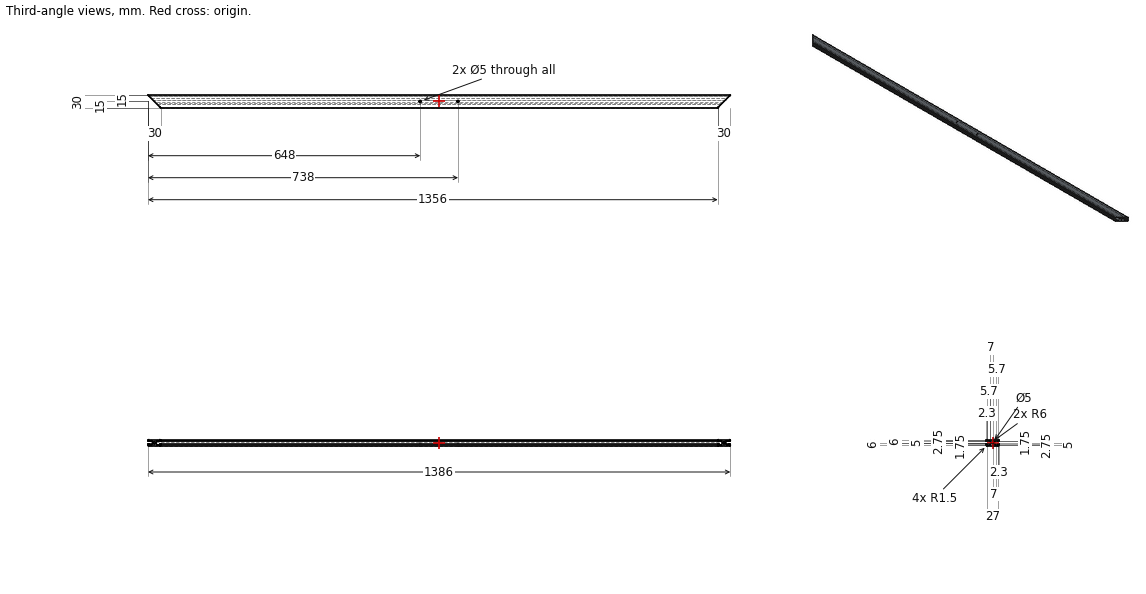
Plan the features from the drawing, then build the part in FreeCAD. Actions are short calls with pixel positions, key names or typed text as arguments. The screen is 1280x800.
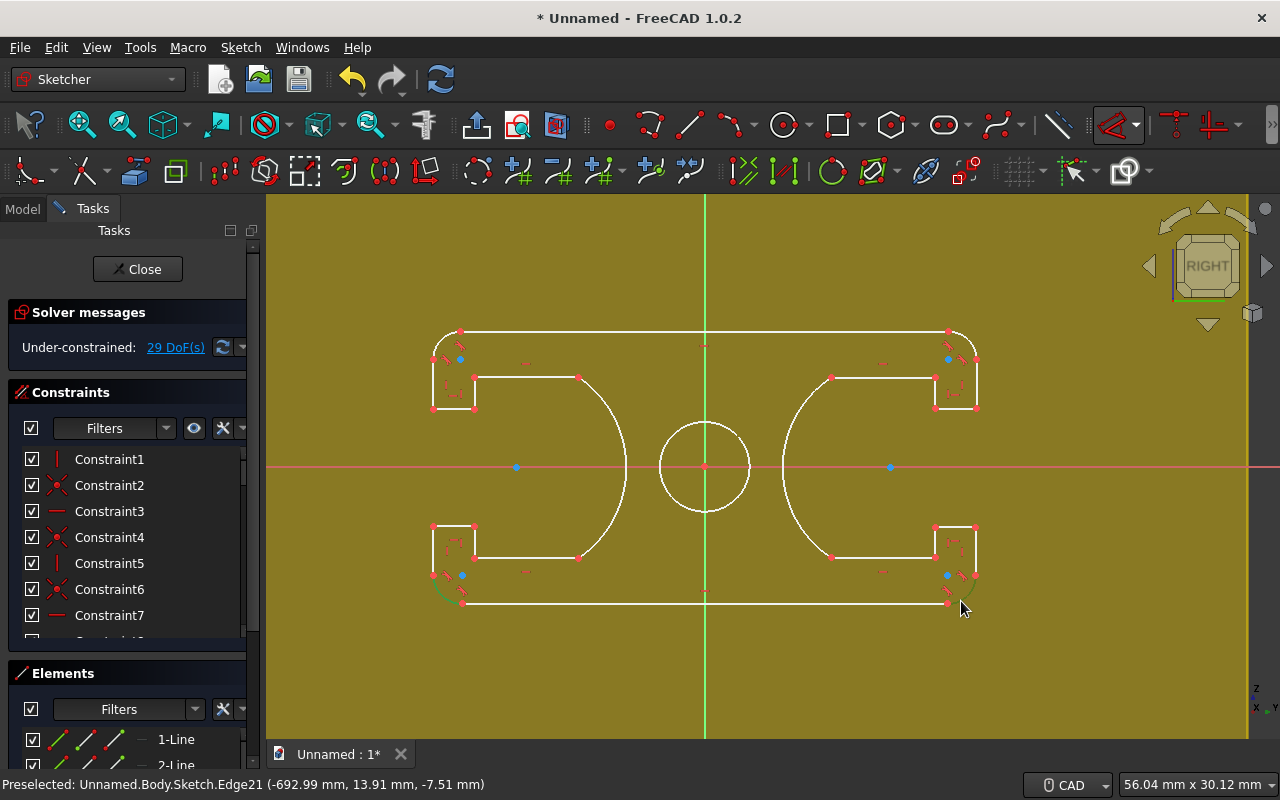
click(973, 347)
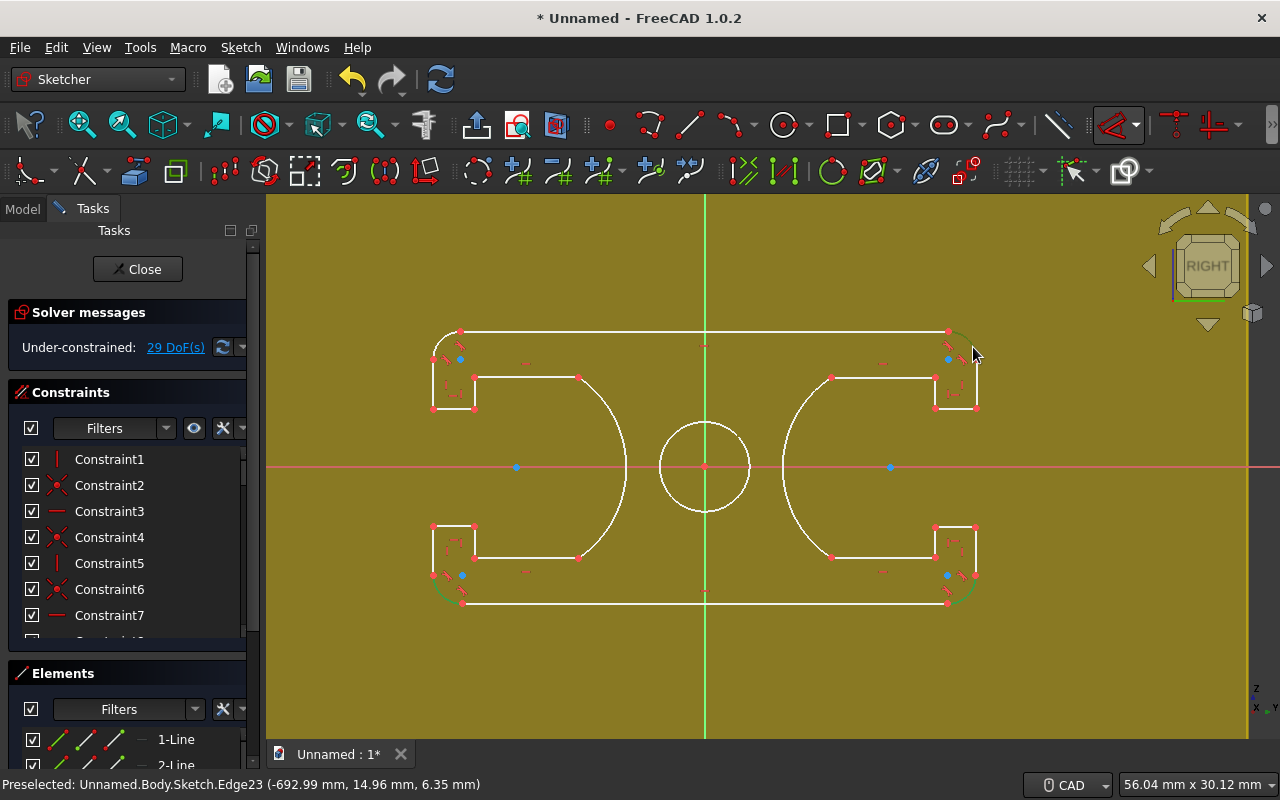
click(448, 335)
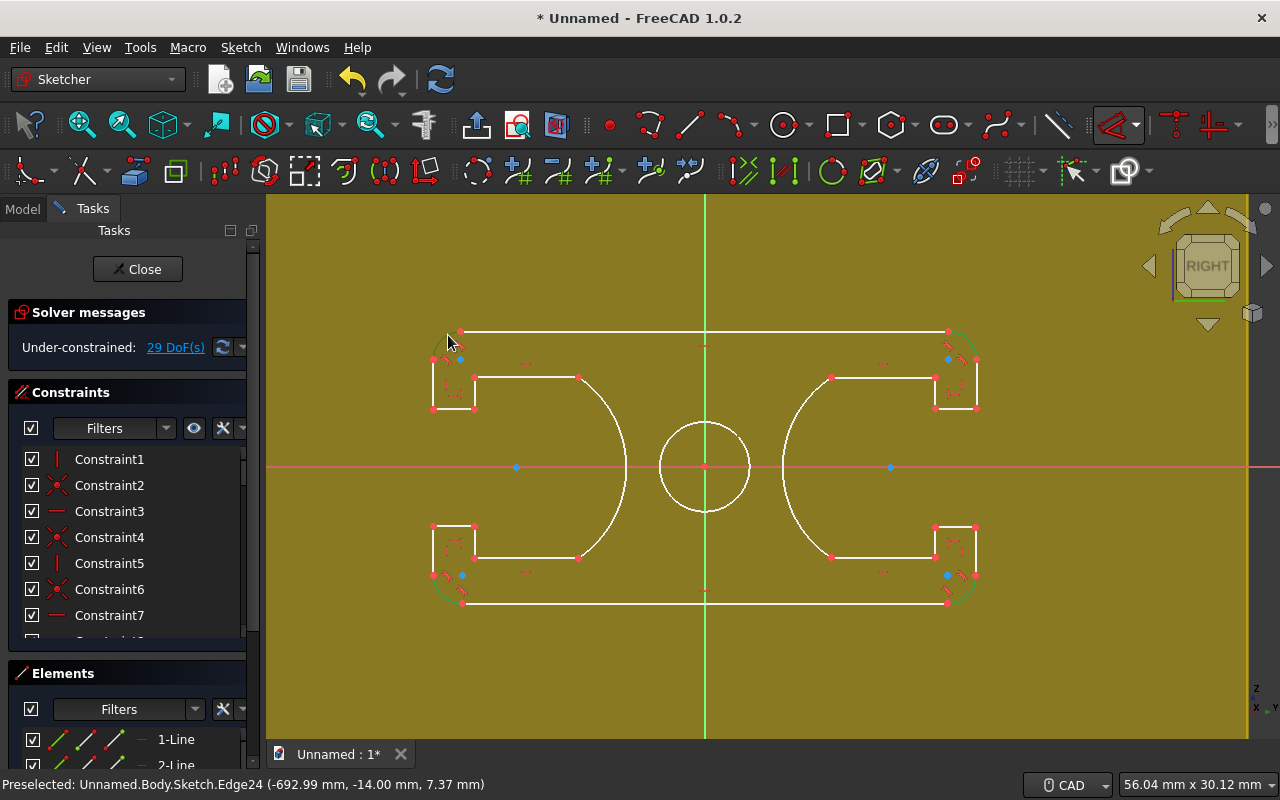
key(e)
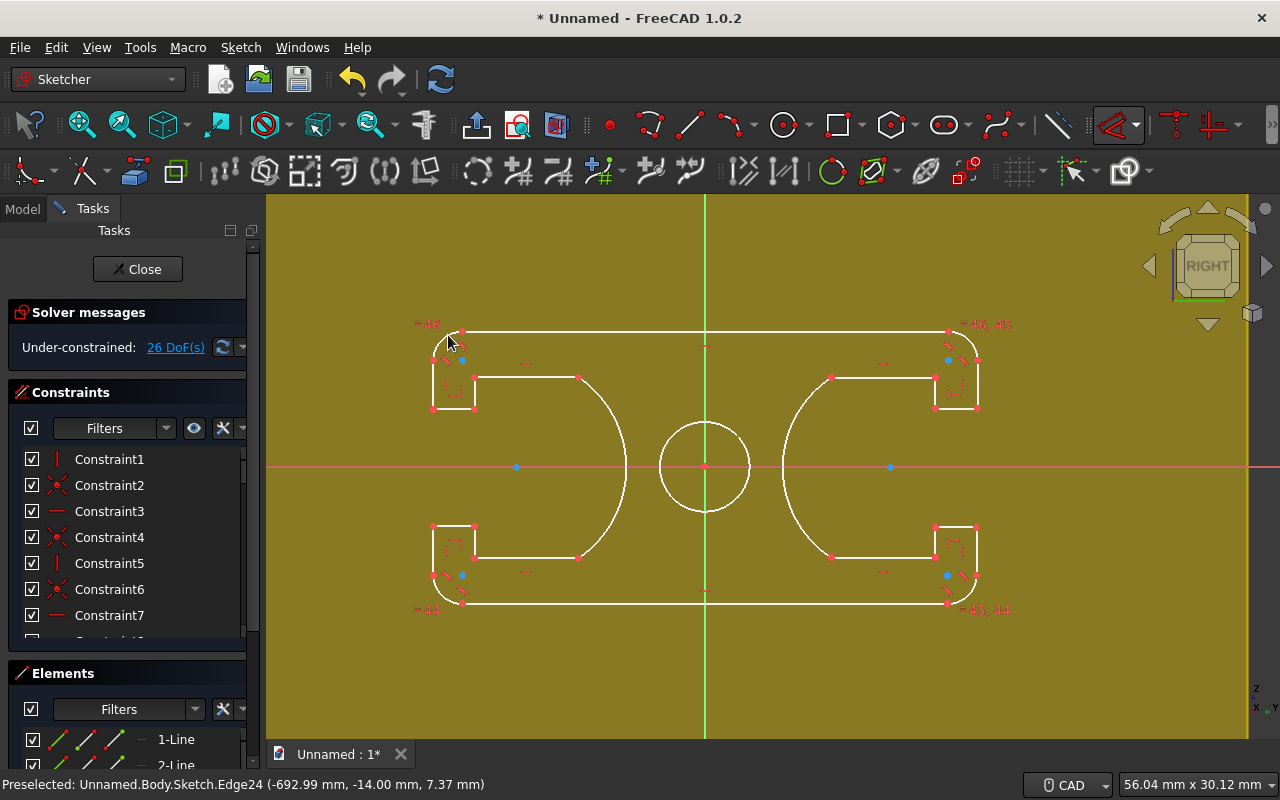
click(618, 509)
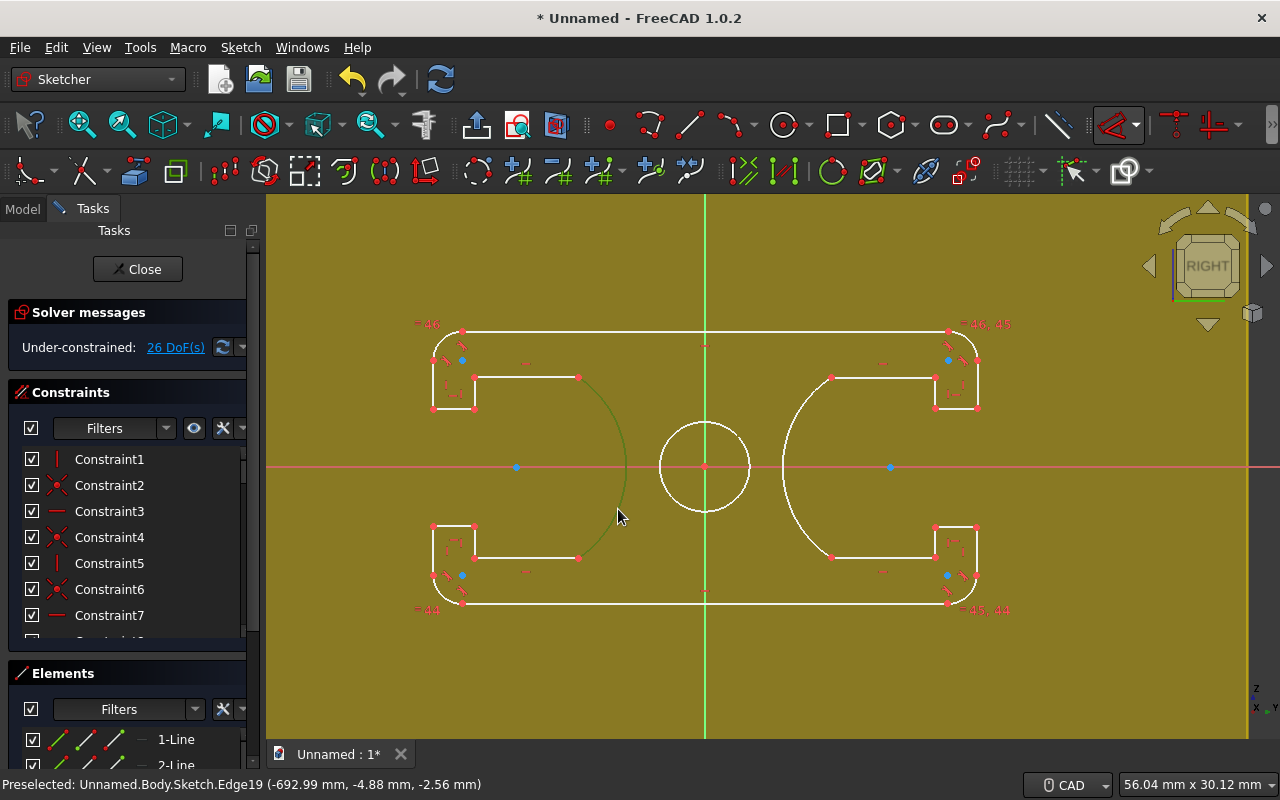
click(791, 426)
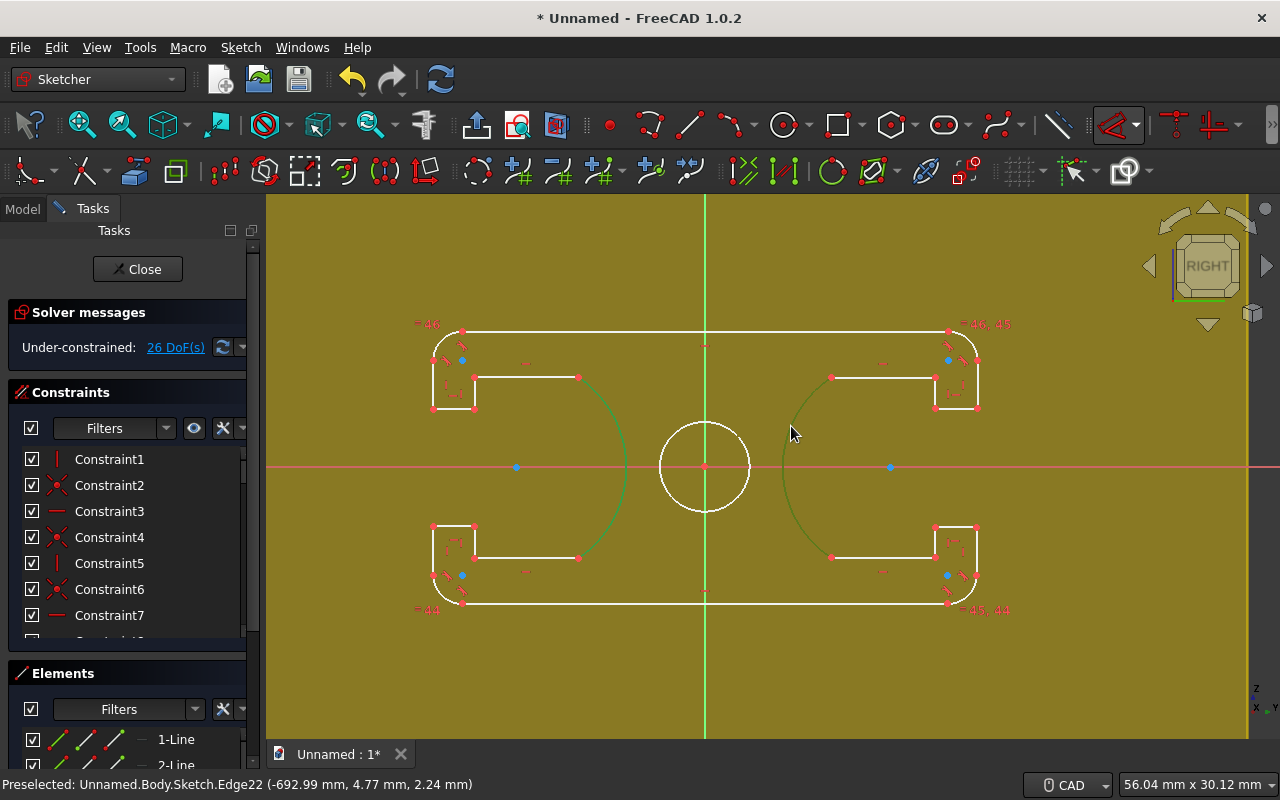
key(e)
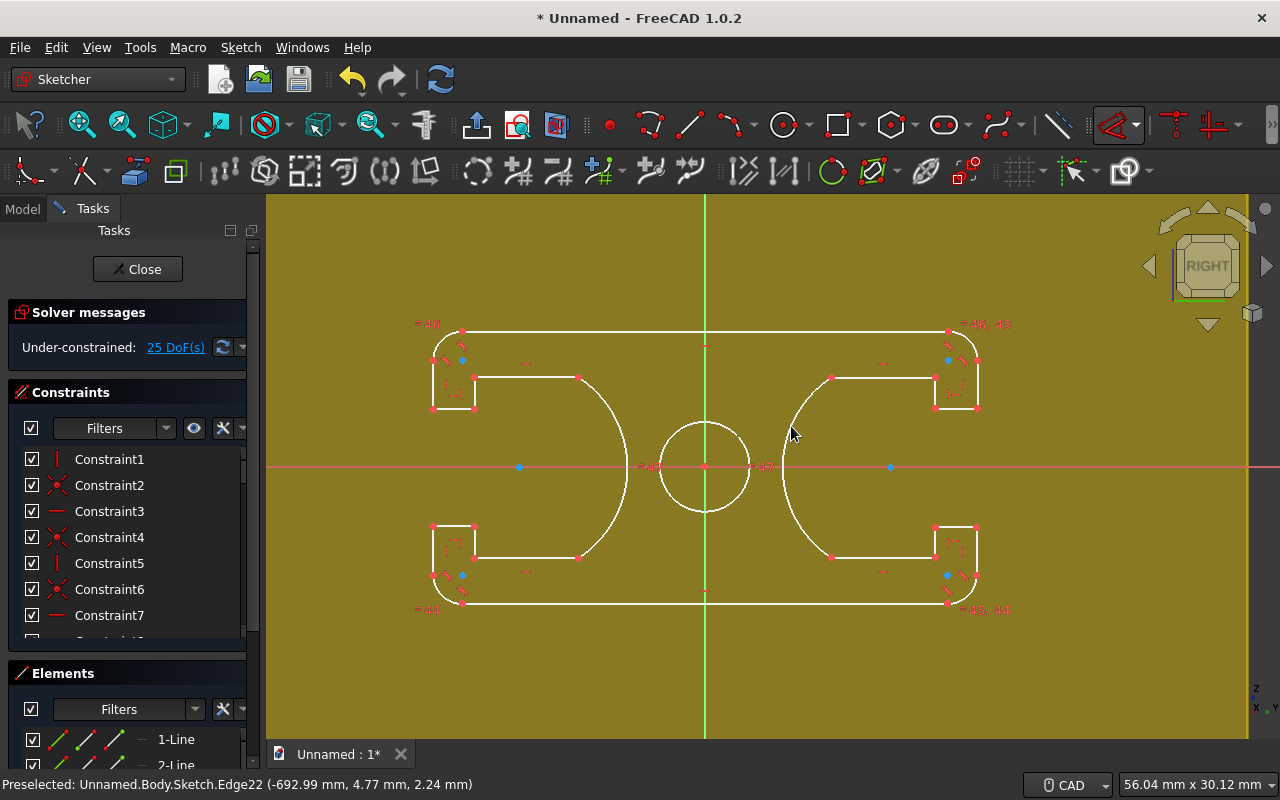
click(519, 468)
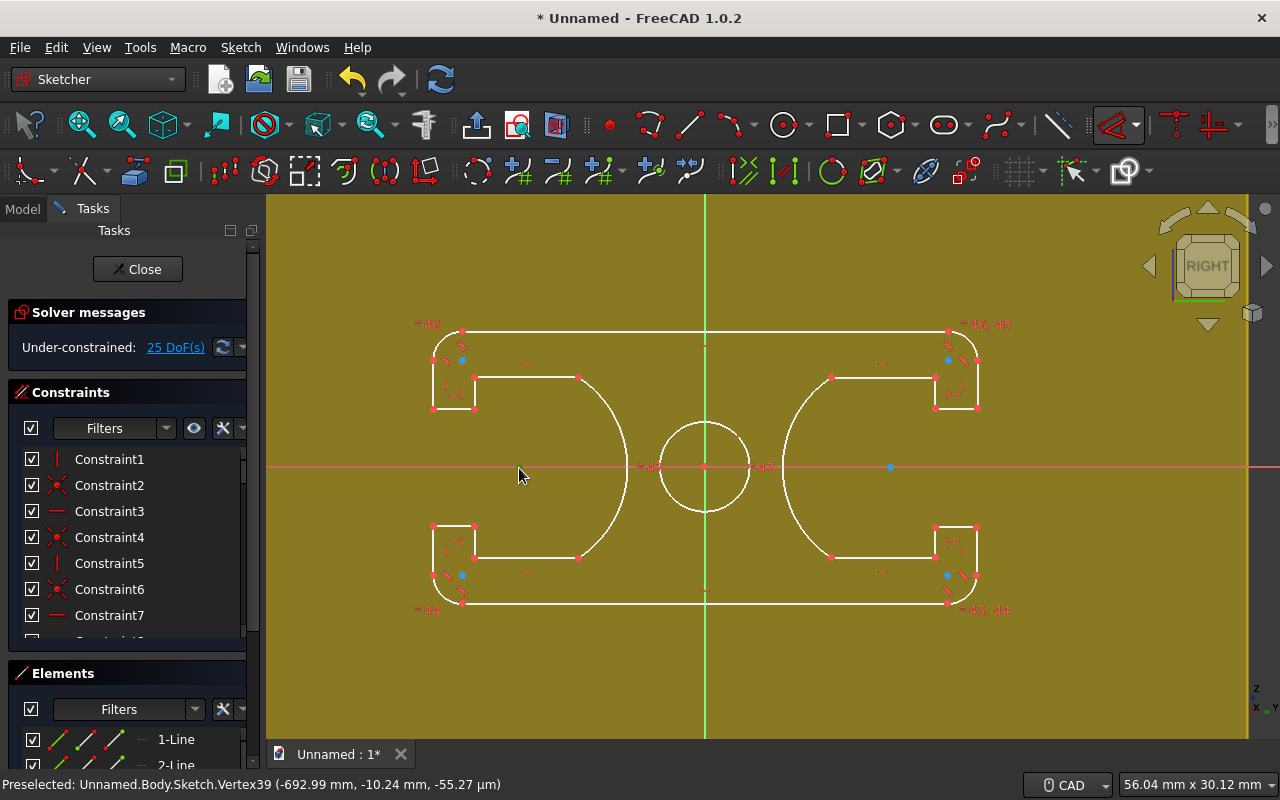
click(353, 467)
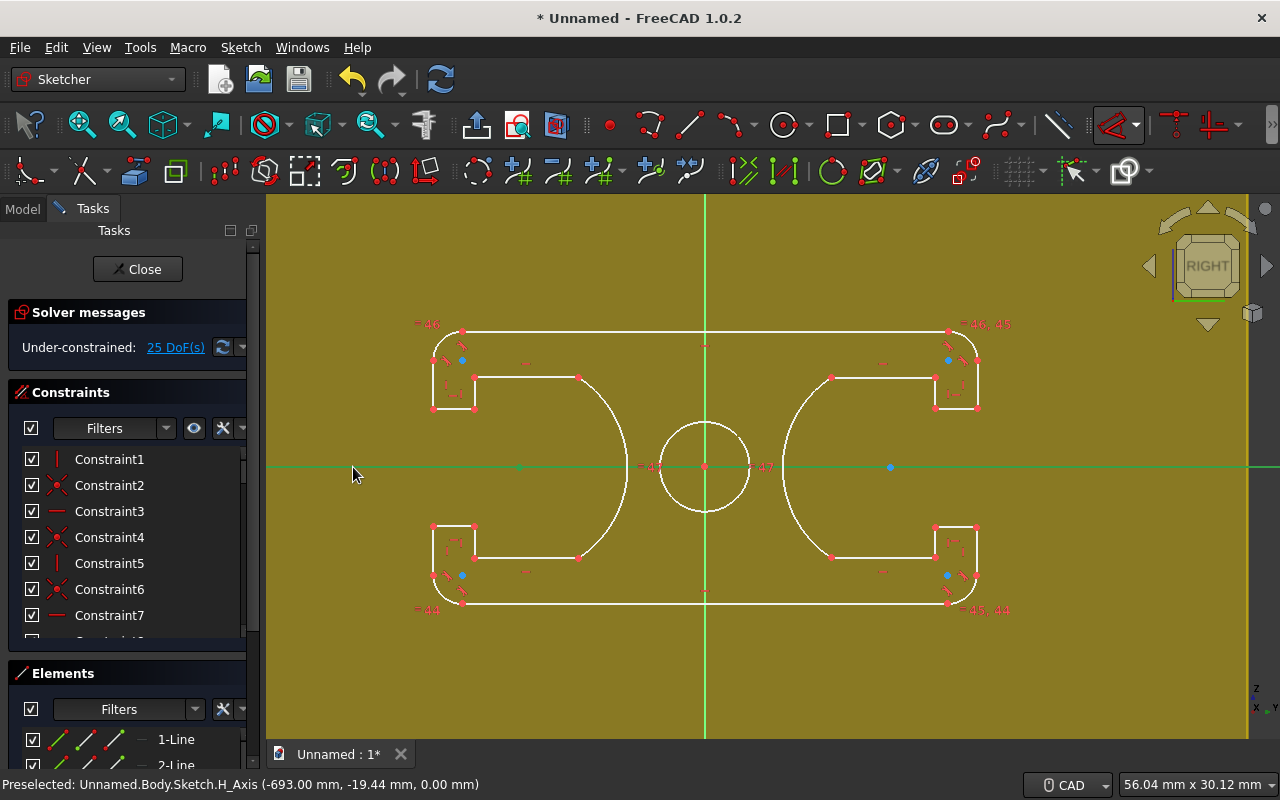
click(1174, 126)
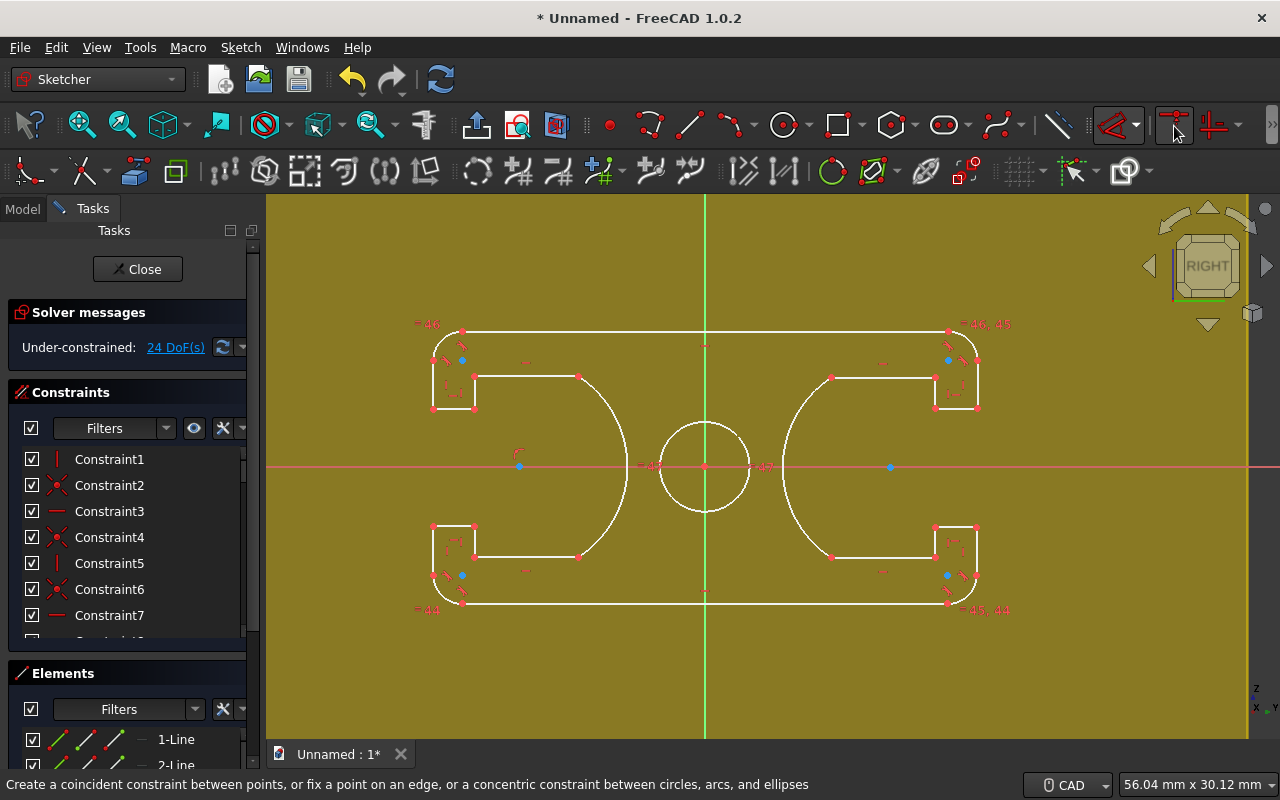
click(891, 468)